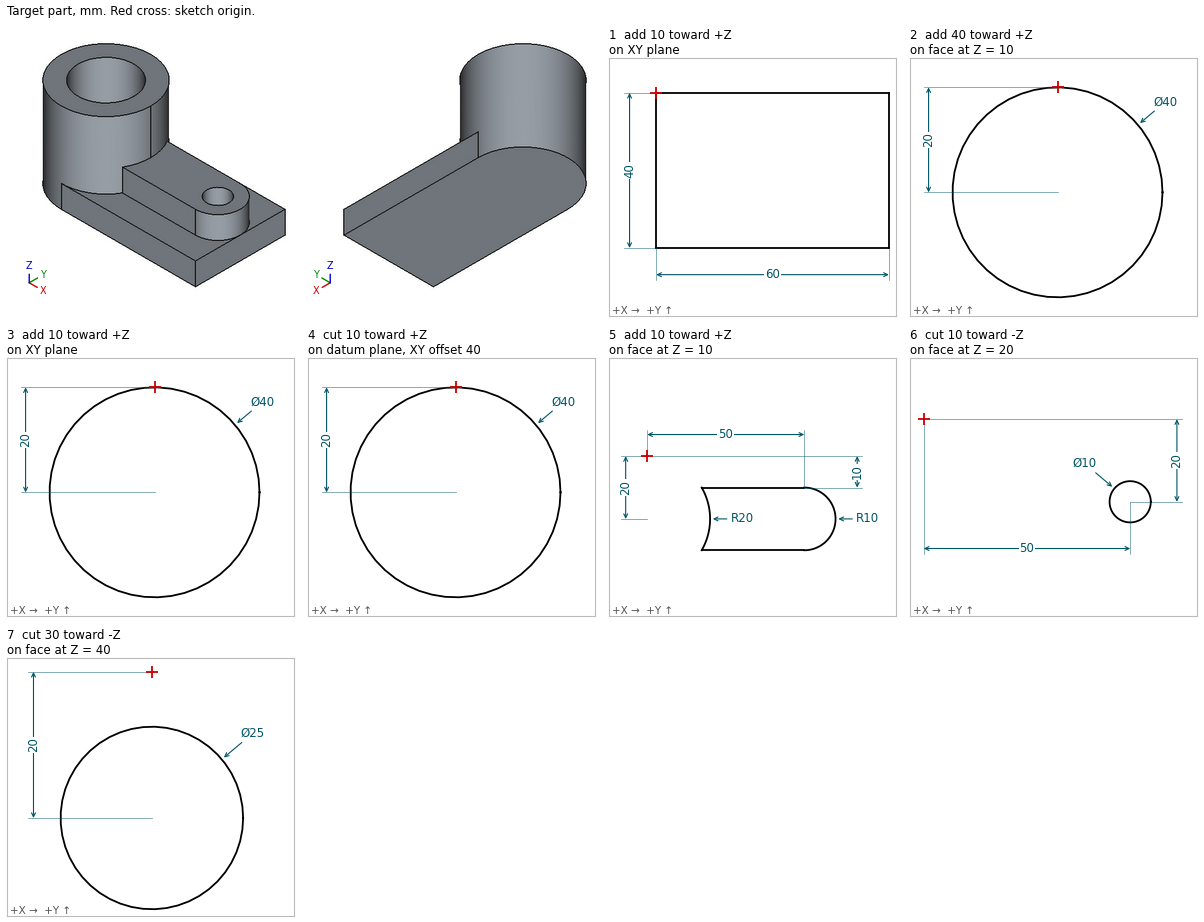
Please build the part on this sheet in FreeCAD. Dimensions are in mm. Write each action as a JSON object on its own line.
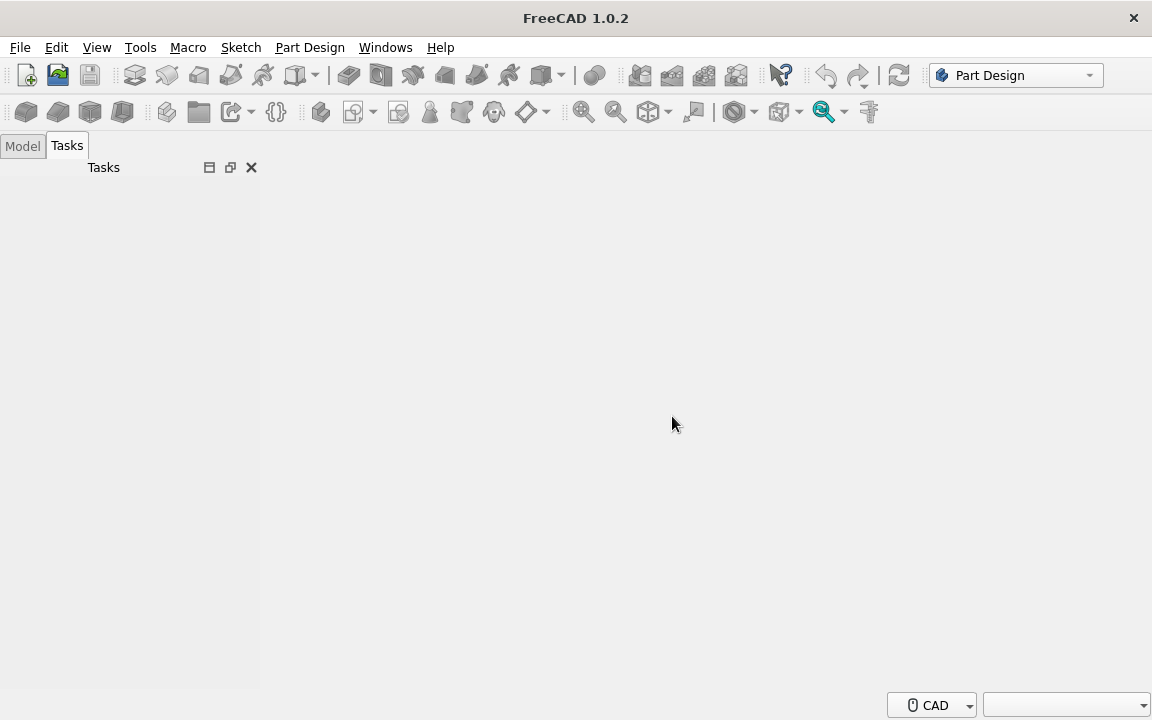
{"action": "left_click", "coordinate": [26, 76]}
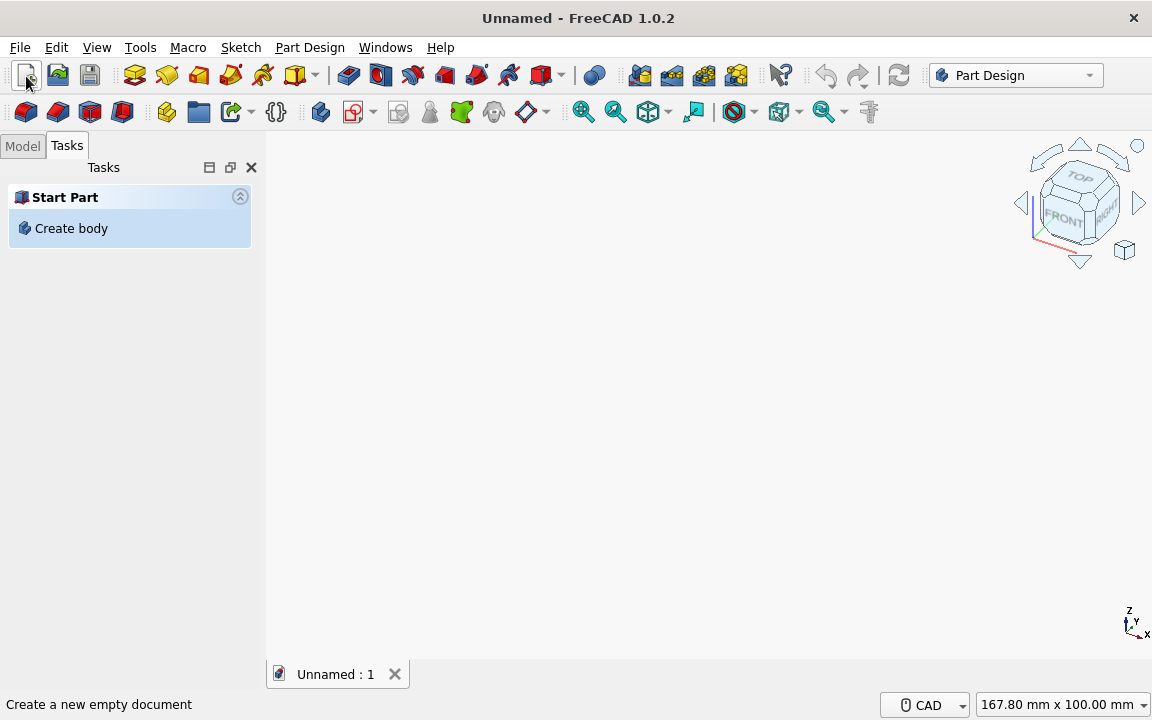
{"action": "left_click", "coordinate": [354, 112]}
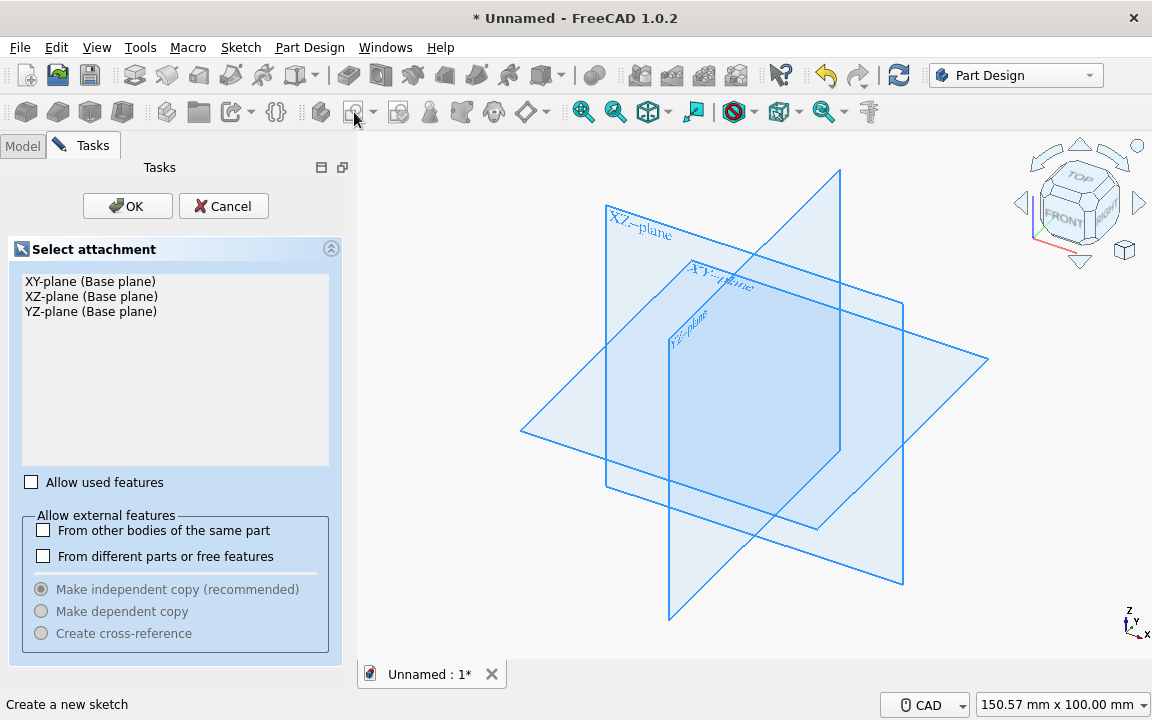
{"action": "left_click", "coordinate": [82, 282]}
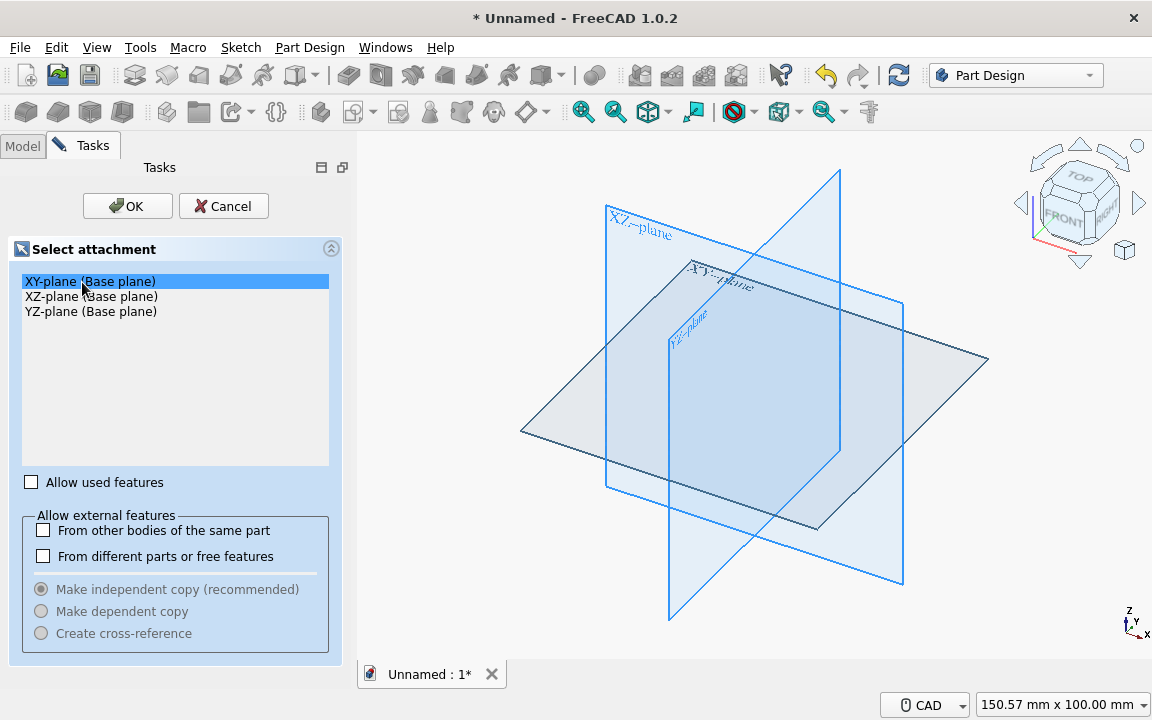
{"action": "left_click", "coordinate": [128, 206]}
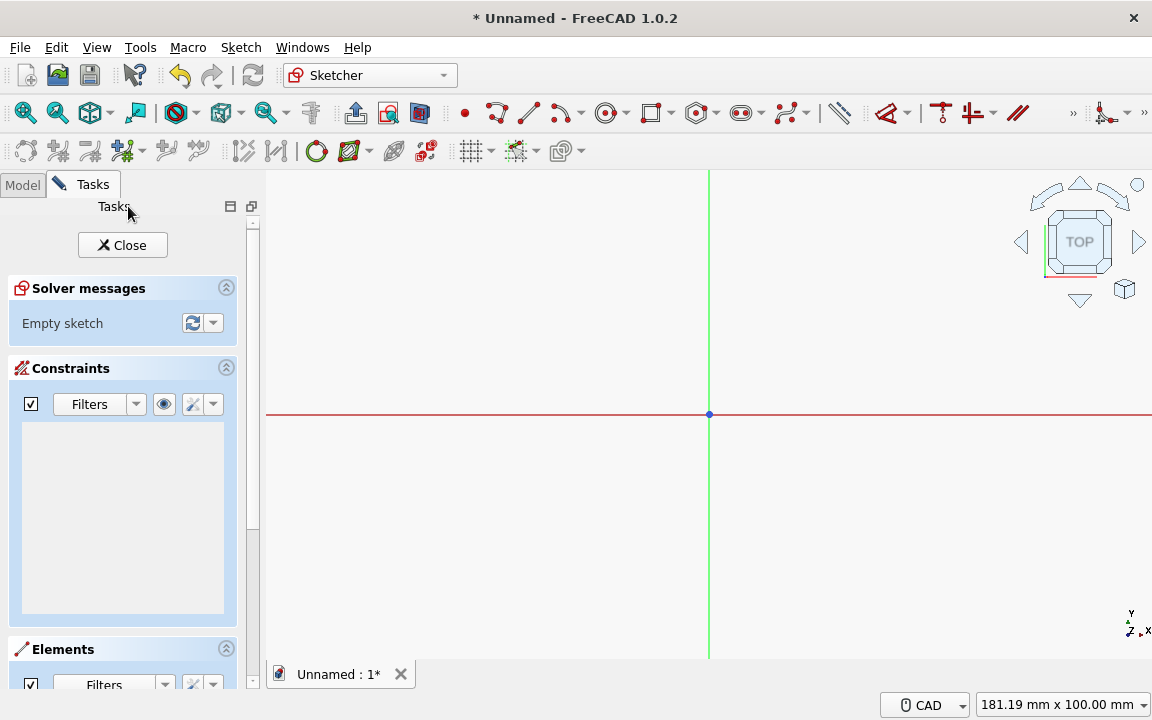
{"action": "scroll", "coordinate": [294, 198], "scroll_direction": "down", "scroll_amount": 1}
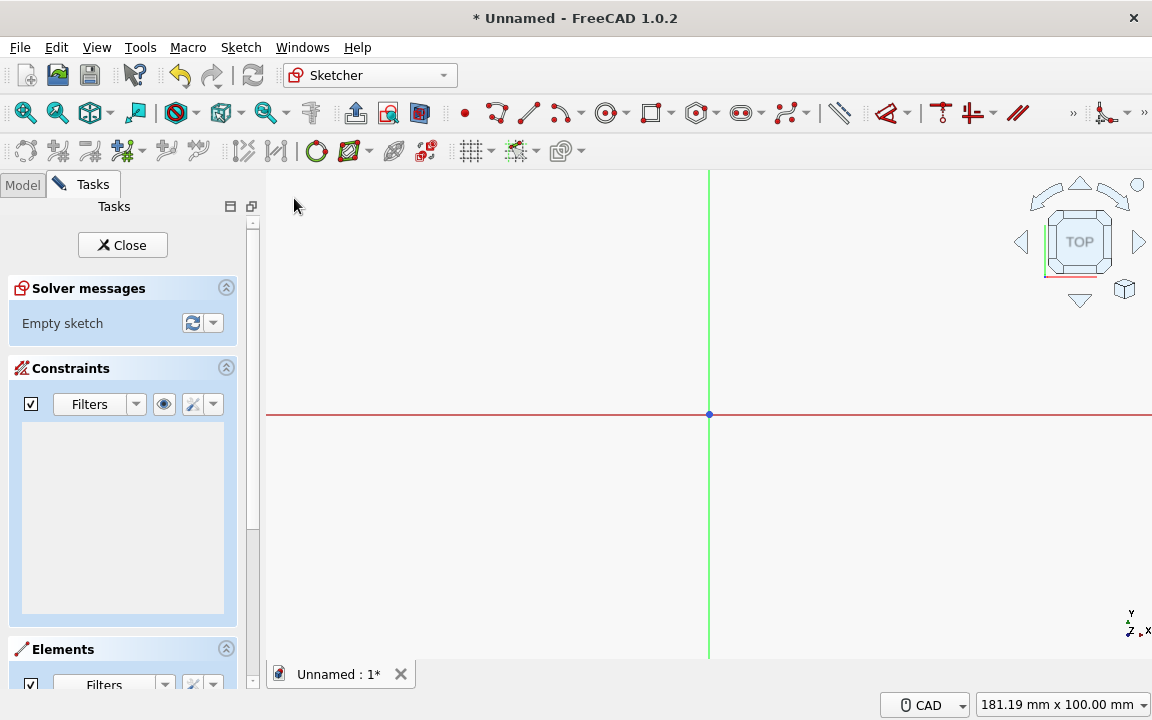
{"action": "scroll", "coordinate": [892, 505], "scroll_direction": "up", "scroll_amount": 3}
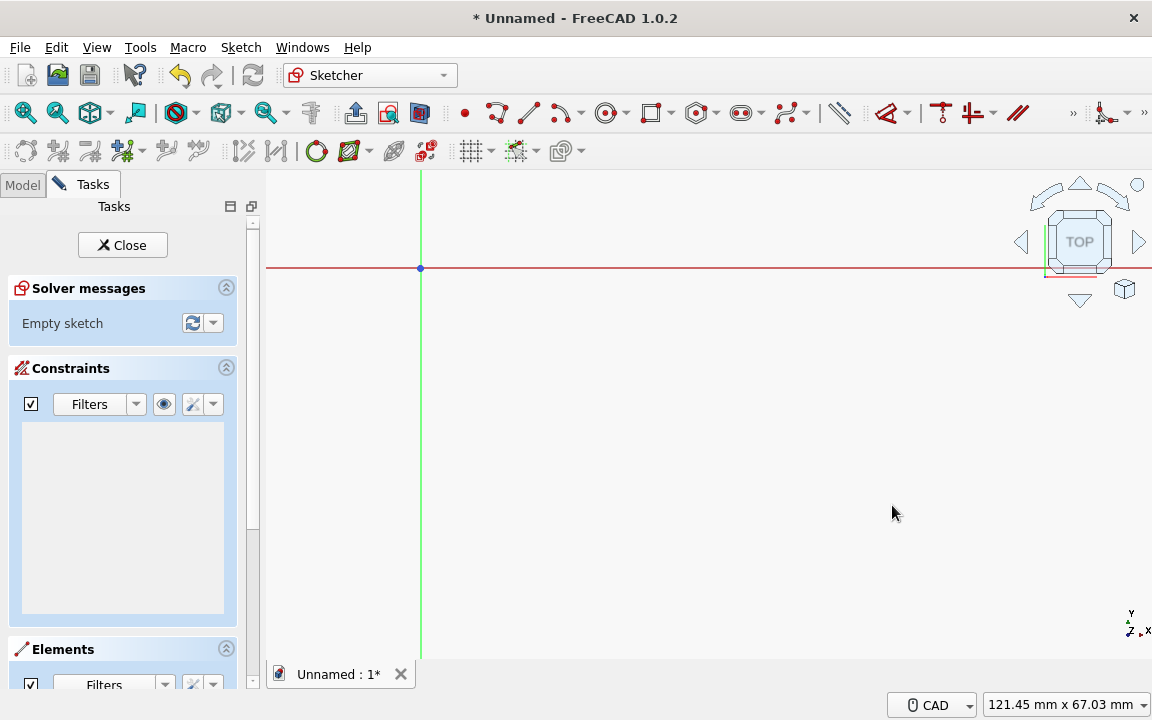
{"action": "left_click", "coordinate": [652, 114]}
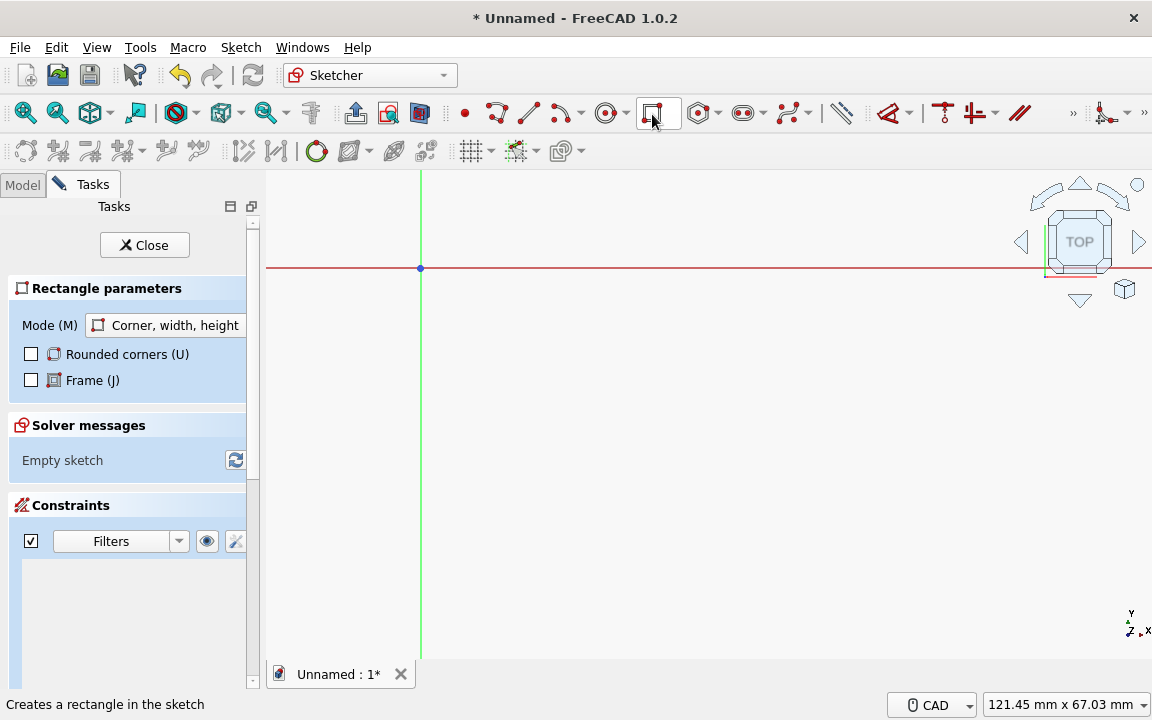
{"action": "left_click", "coordinate": [421, 268]}
{"action": "left_click", "coordinate": [859, 560]}
{"action": "key", "text": "Escape"}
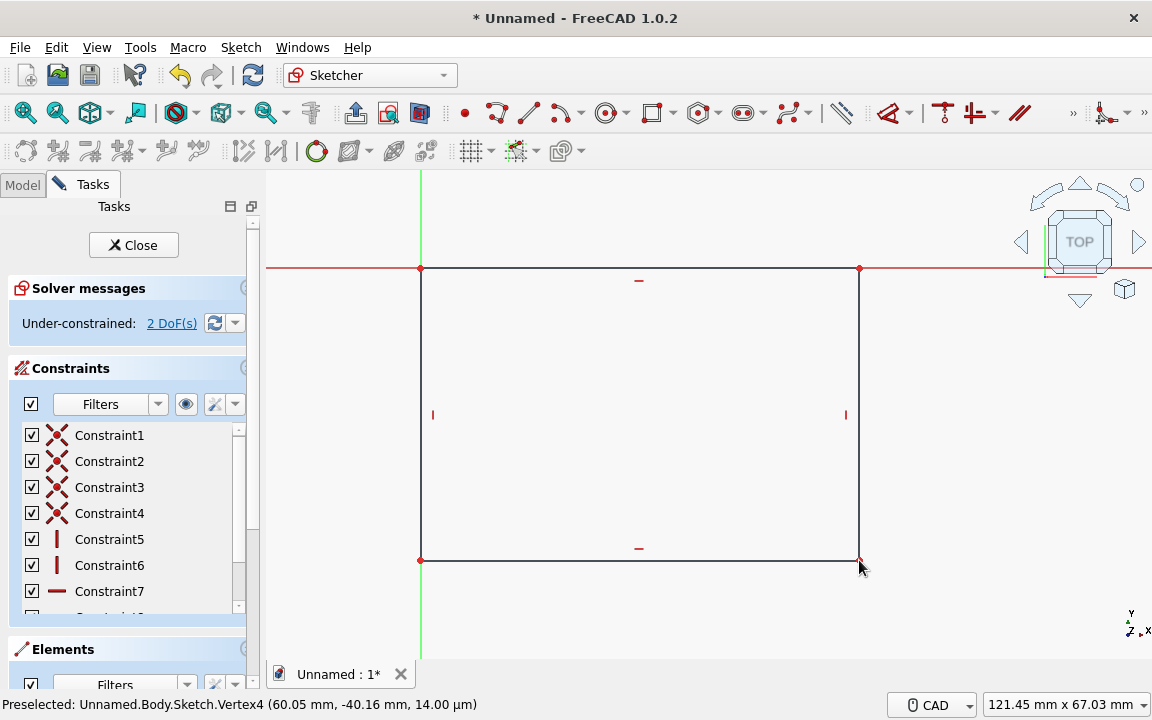
{"action": "left_click", "coordinate": [888, 114]}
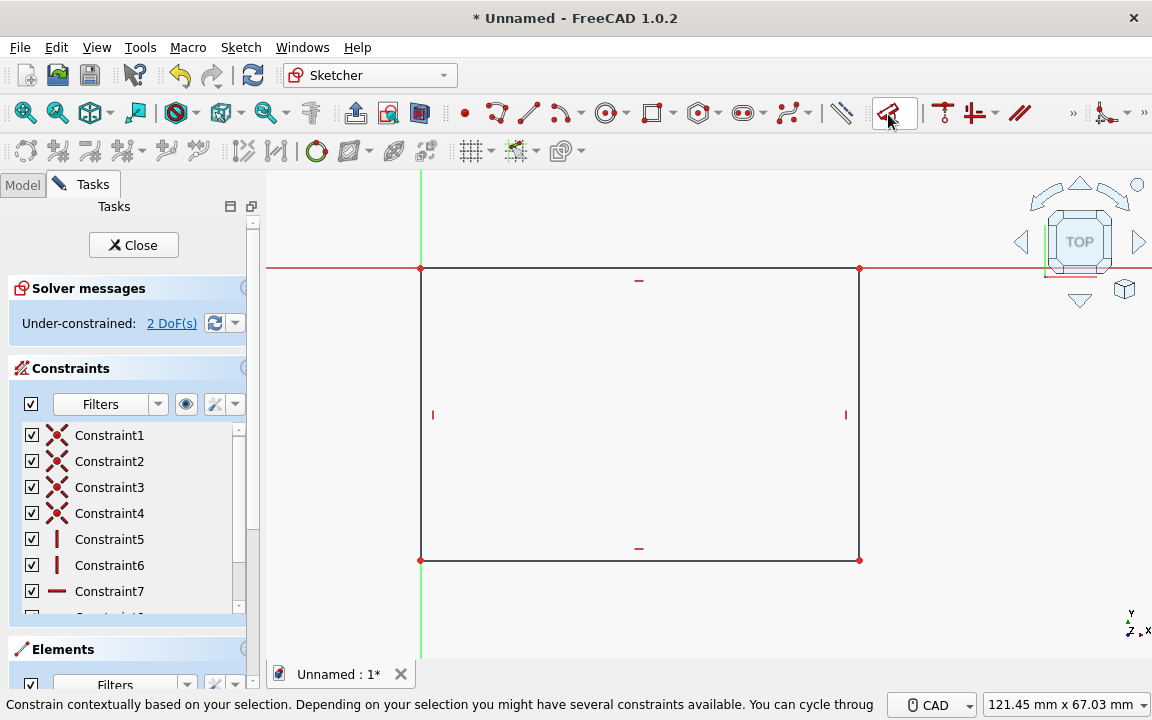
{"action": "left_click", "coordinate": [421, 356]}
{"action": "left_click", "coordinate": [387, 415]}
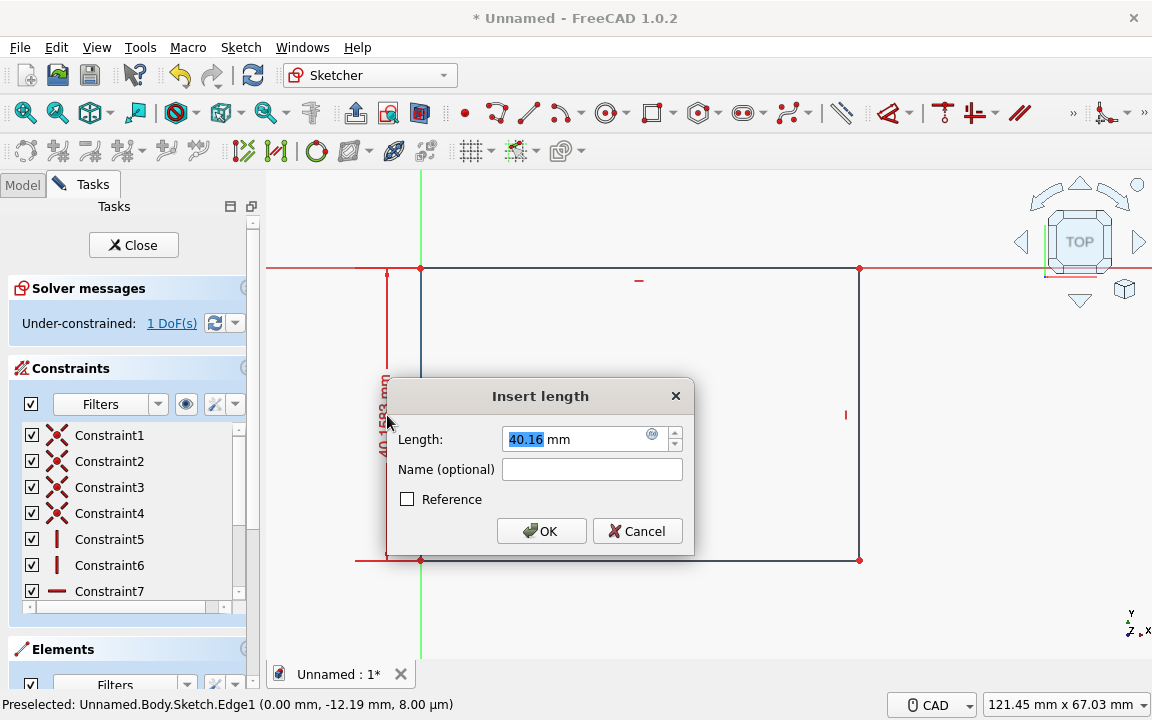
{"action": "type", "text": "40"}
{"action": "key", "text": "Return"}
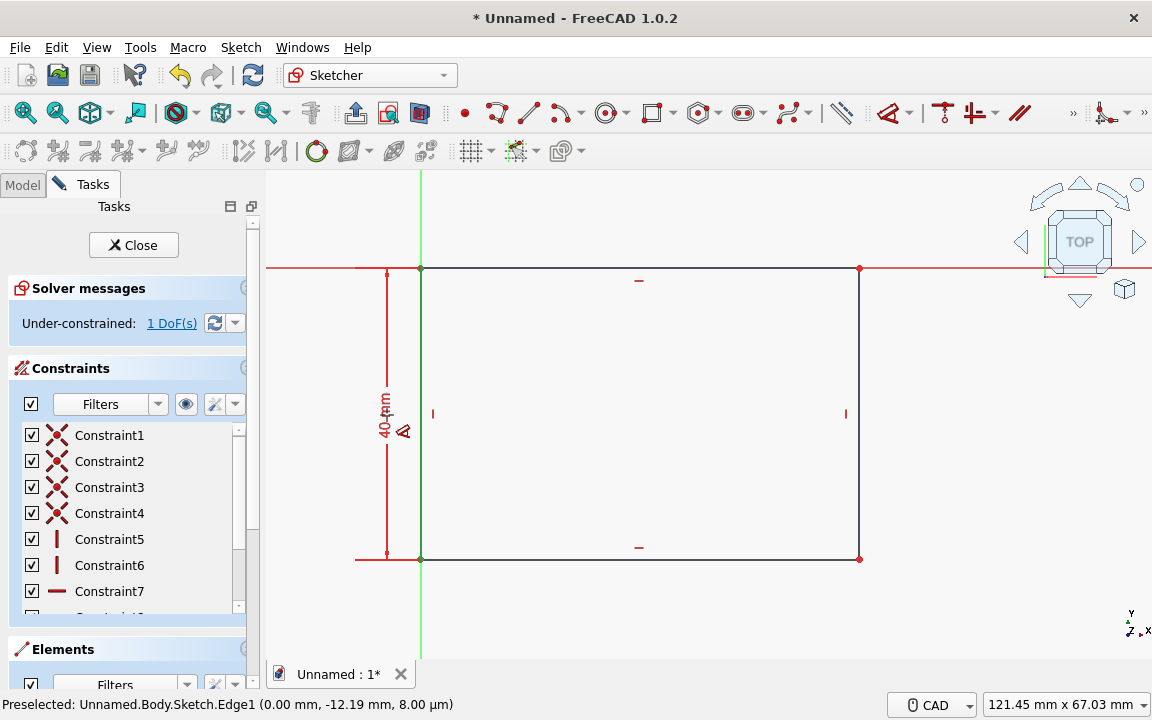
{"action": "left_click", "coordinate": [552, 560]}
{"action": "left_click", "coordinate": [640, 594]}